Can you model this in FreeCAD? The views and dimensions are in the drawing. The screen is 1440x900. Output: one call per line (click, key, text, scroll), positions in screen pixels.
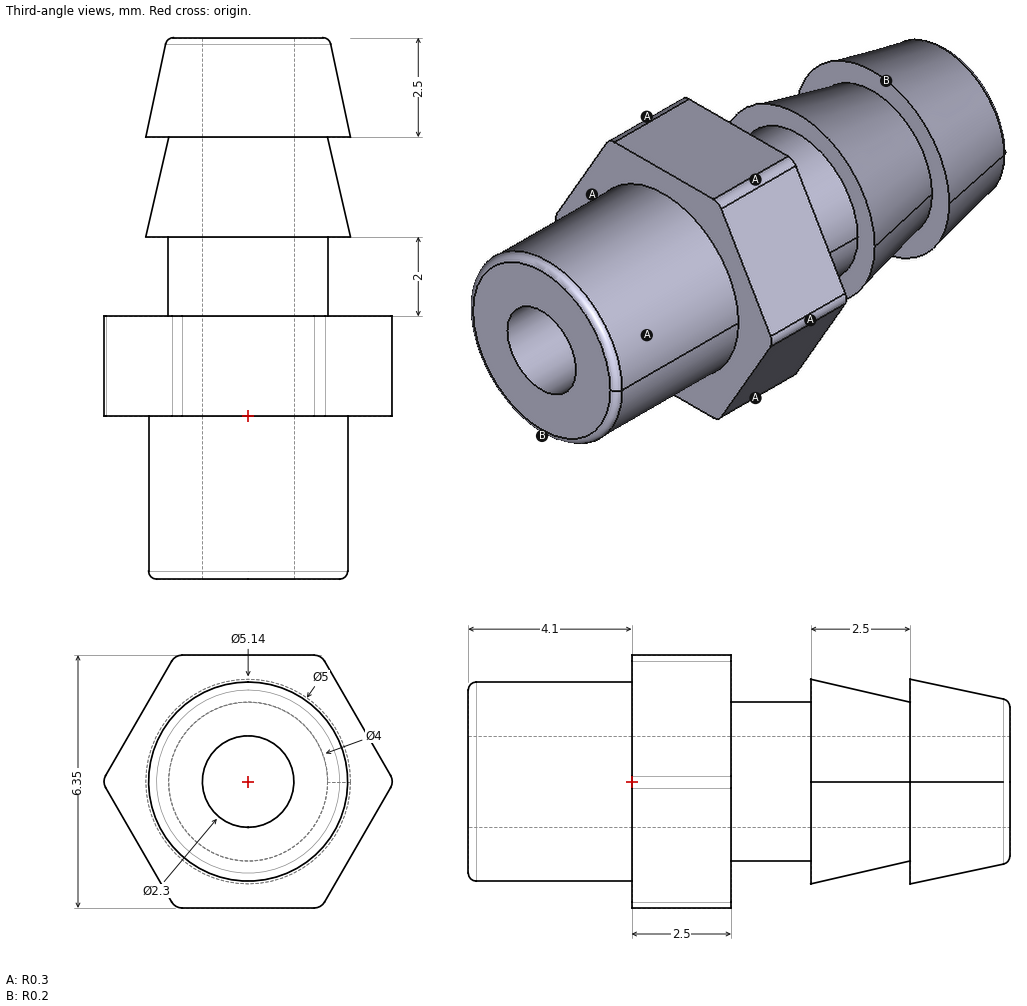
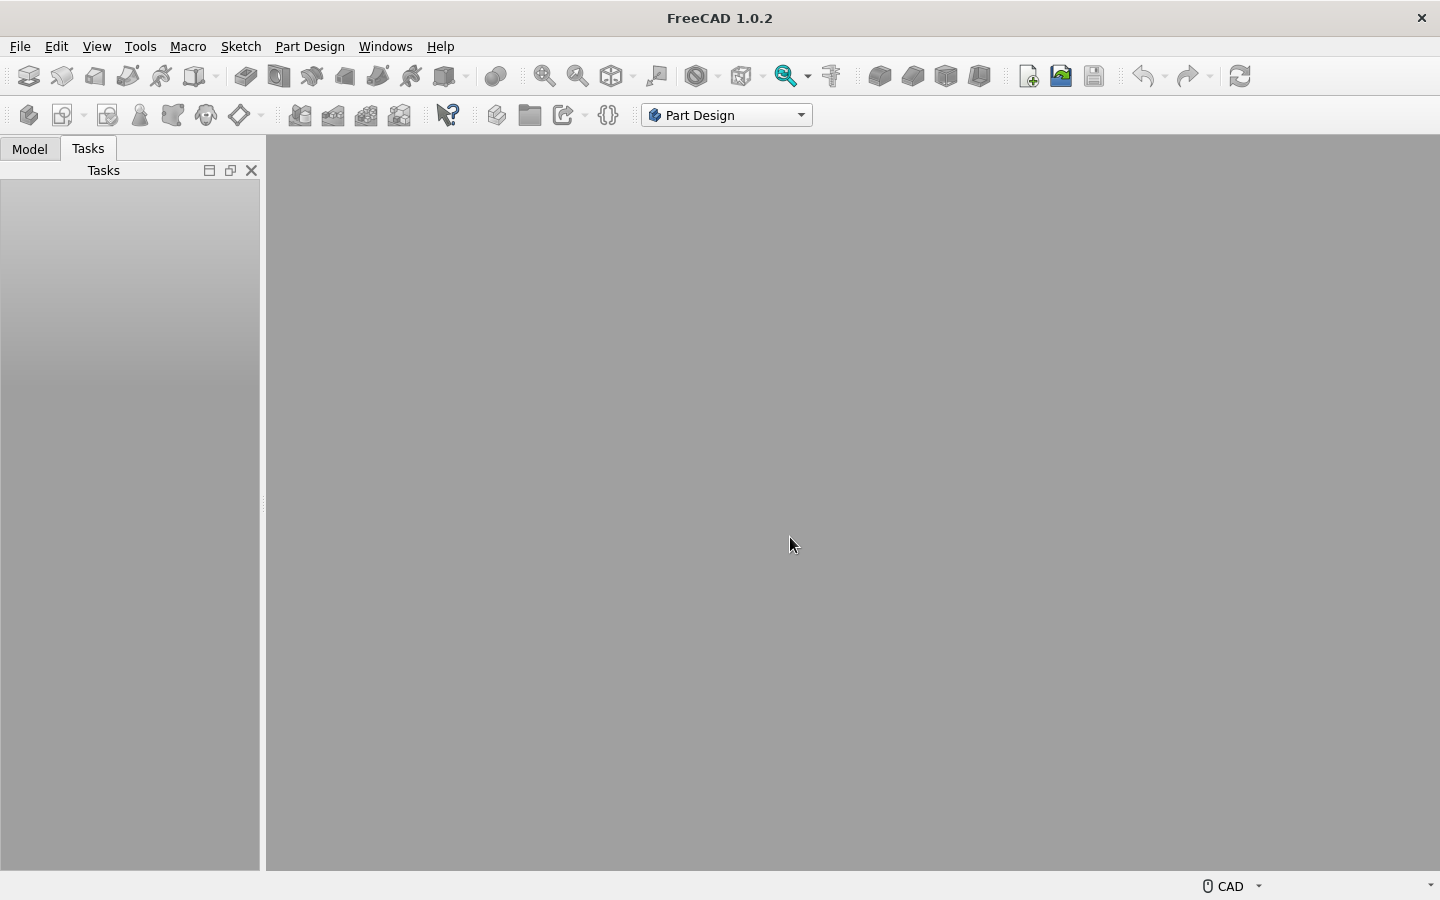
key(ctrl+n)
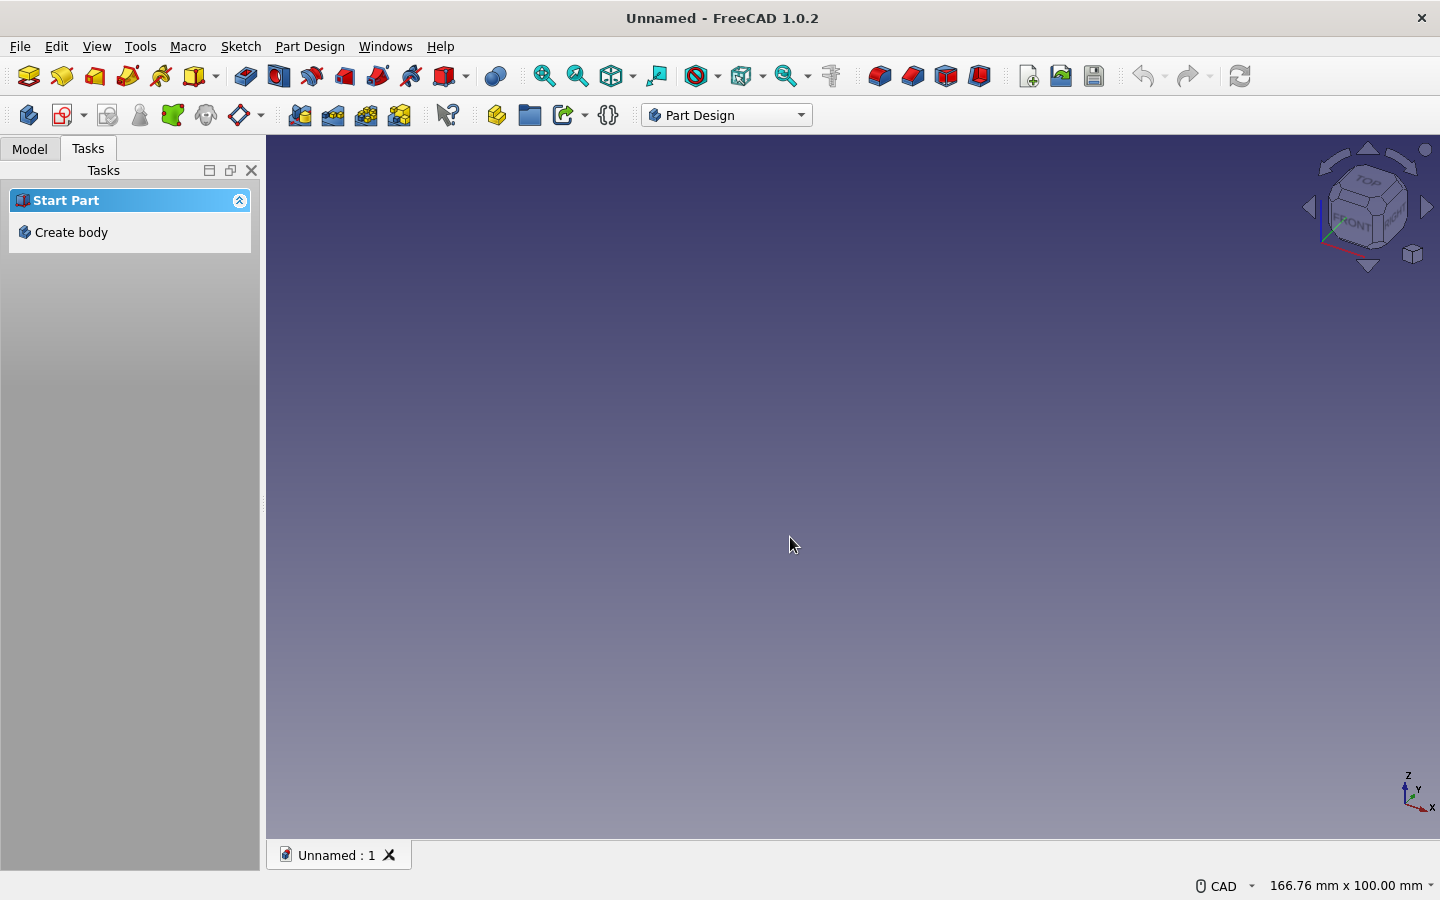
click(62, 116)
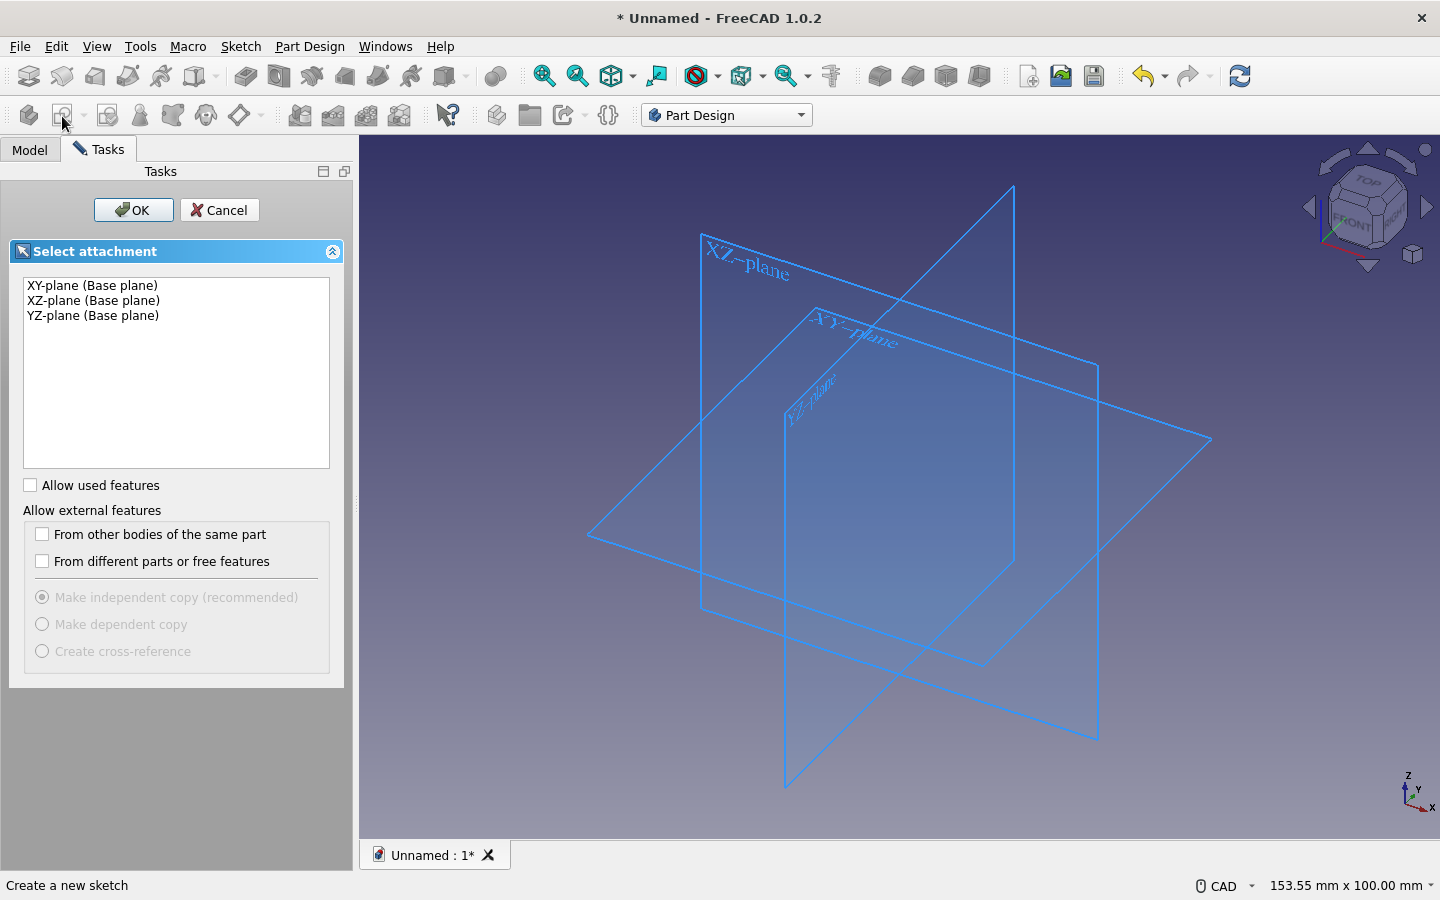
click(84, 300)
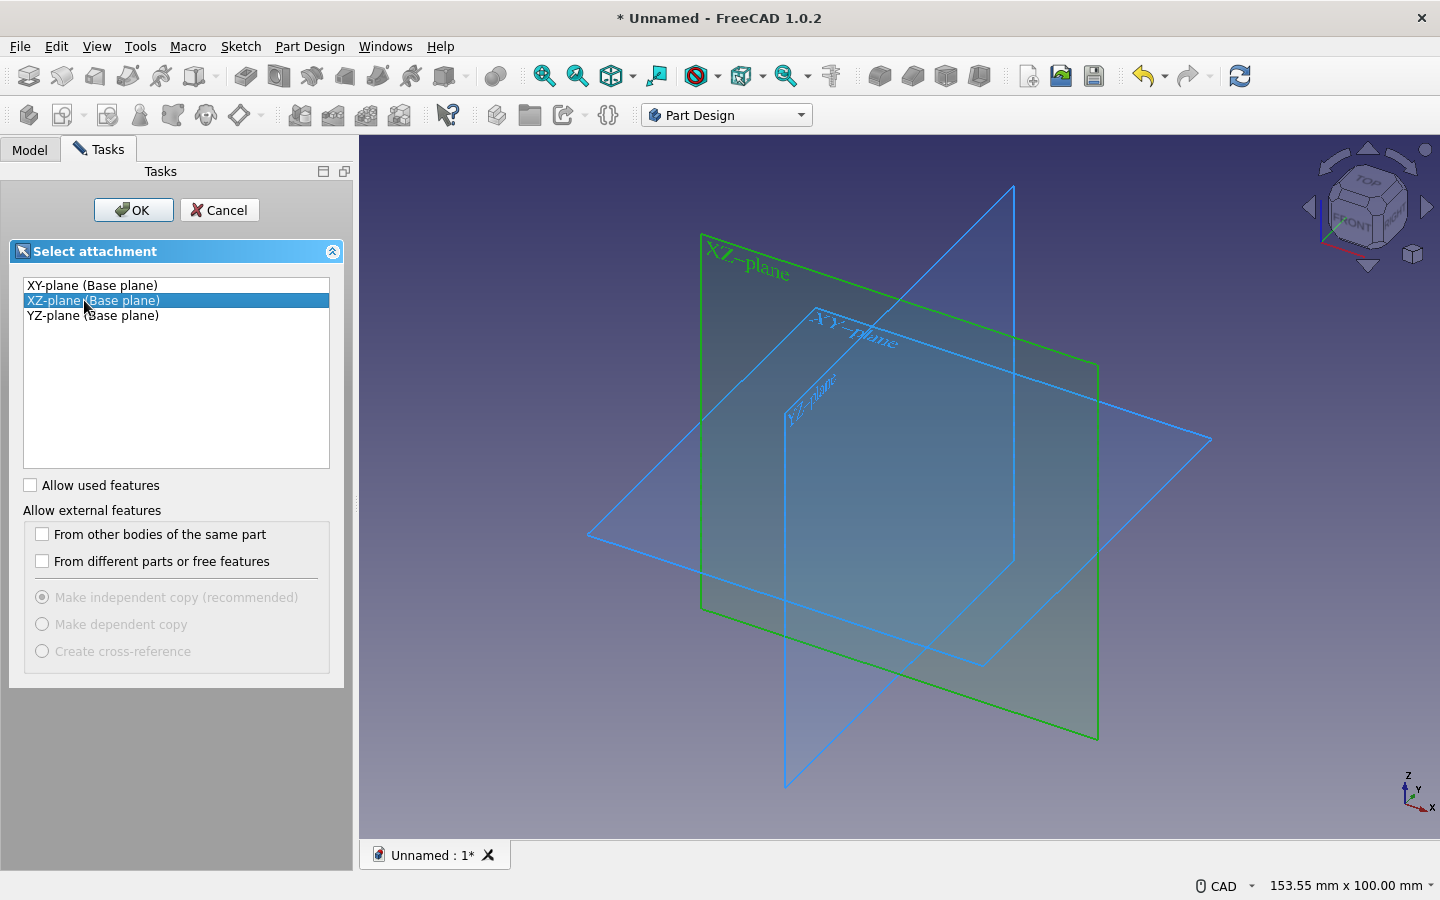
click(134, 210)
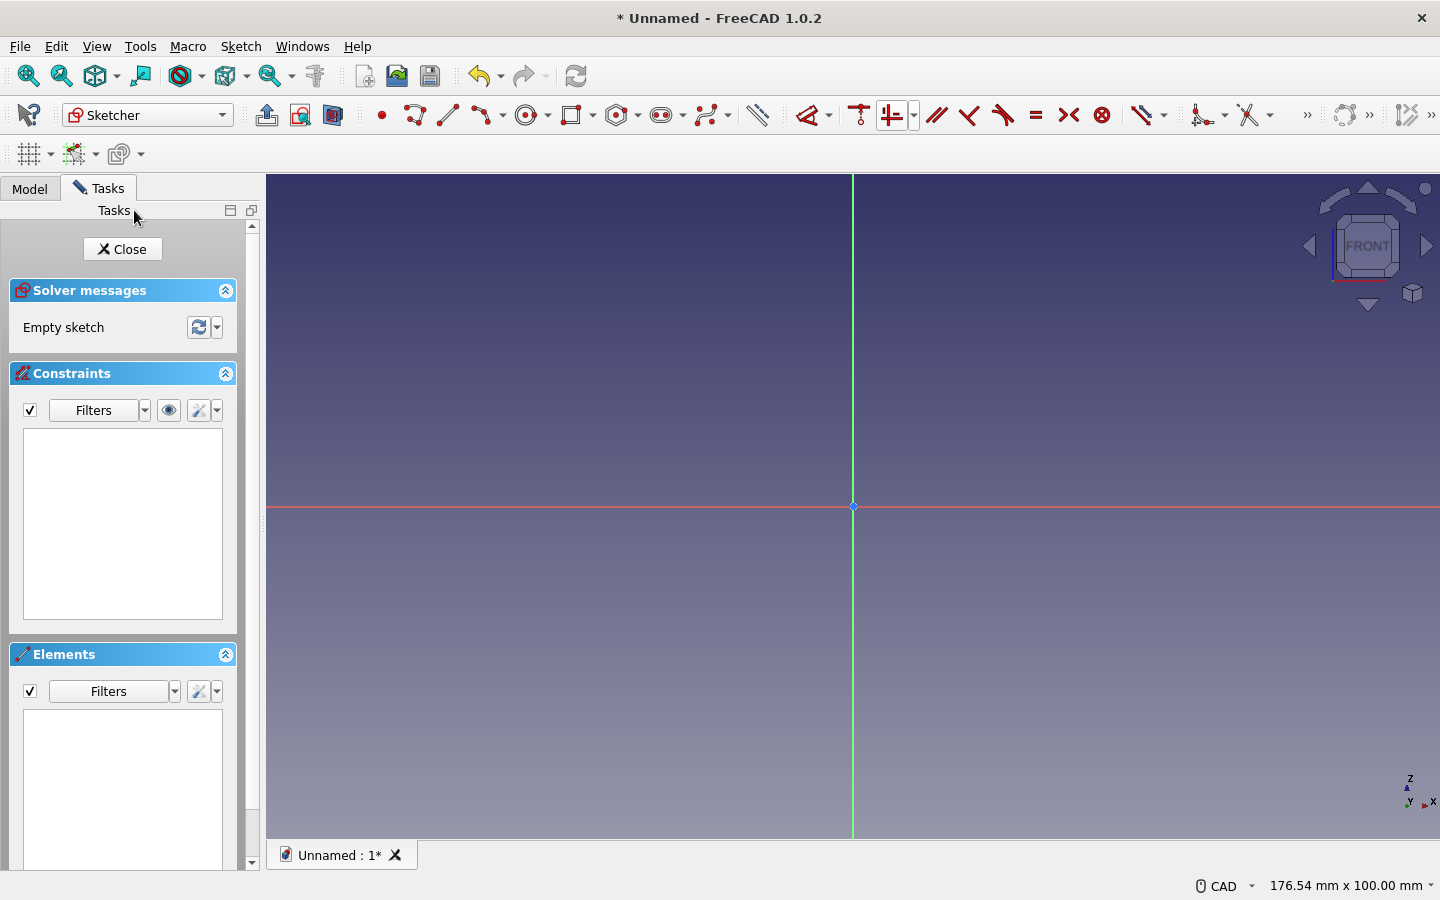
scroll(860, 506, up, 12)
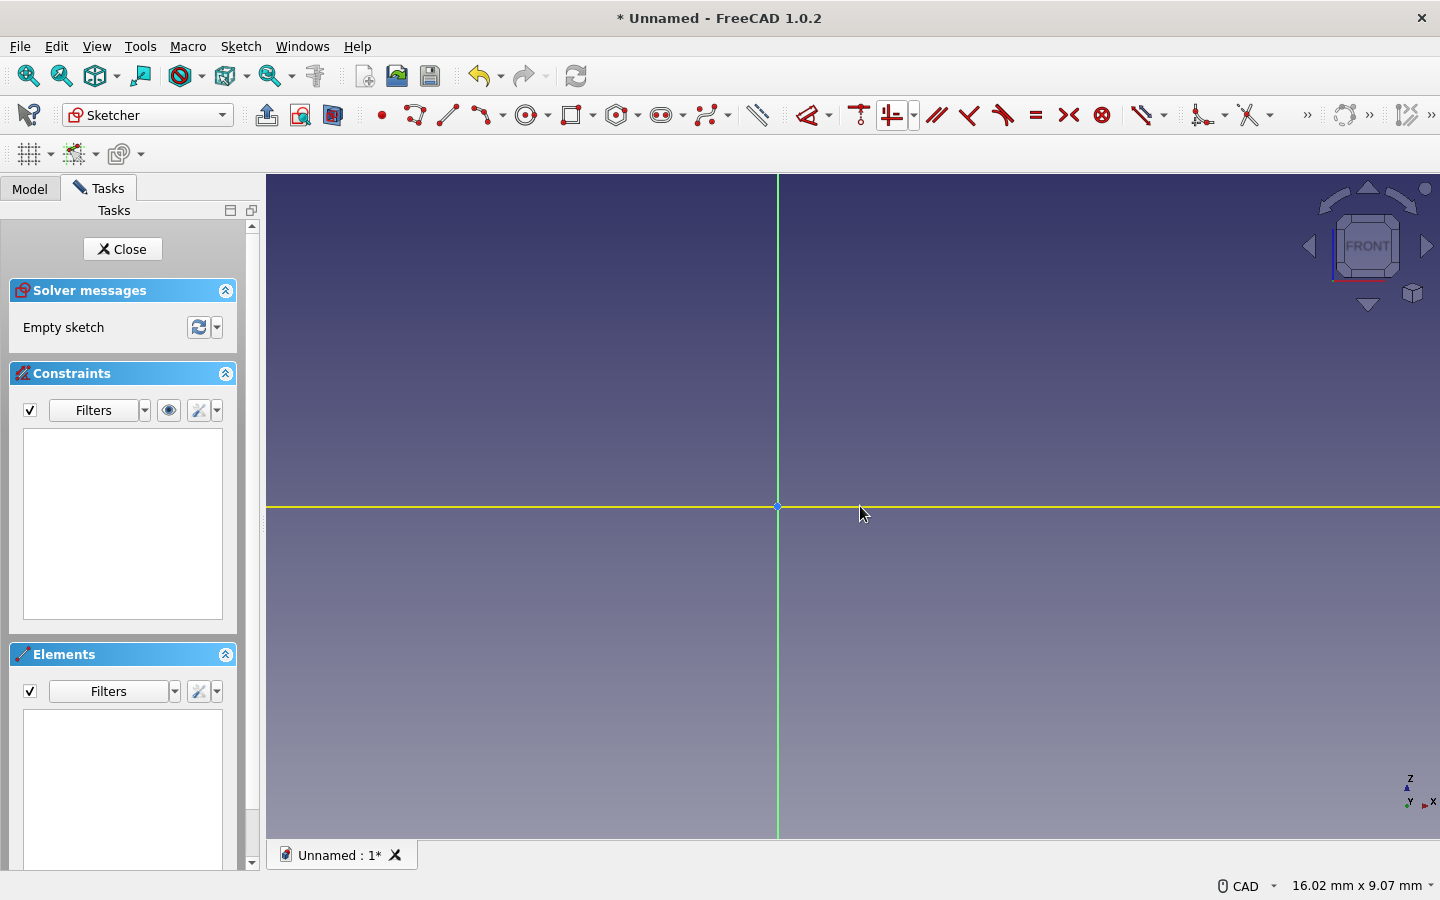
click(616, 116)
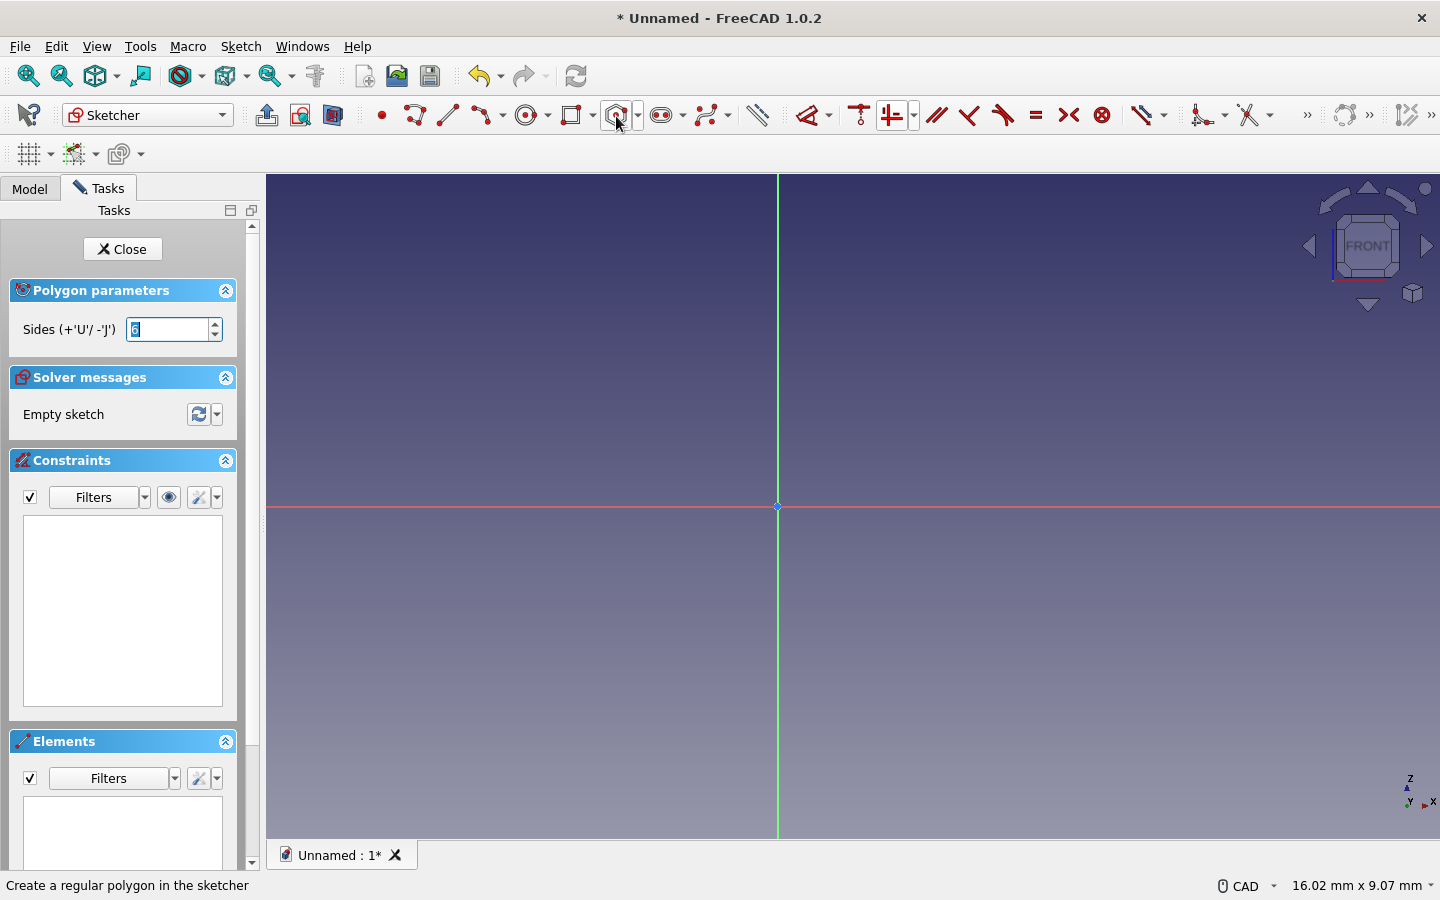
click(778, 506)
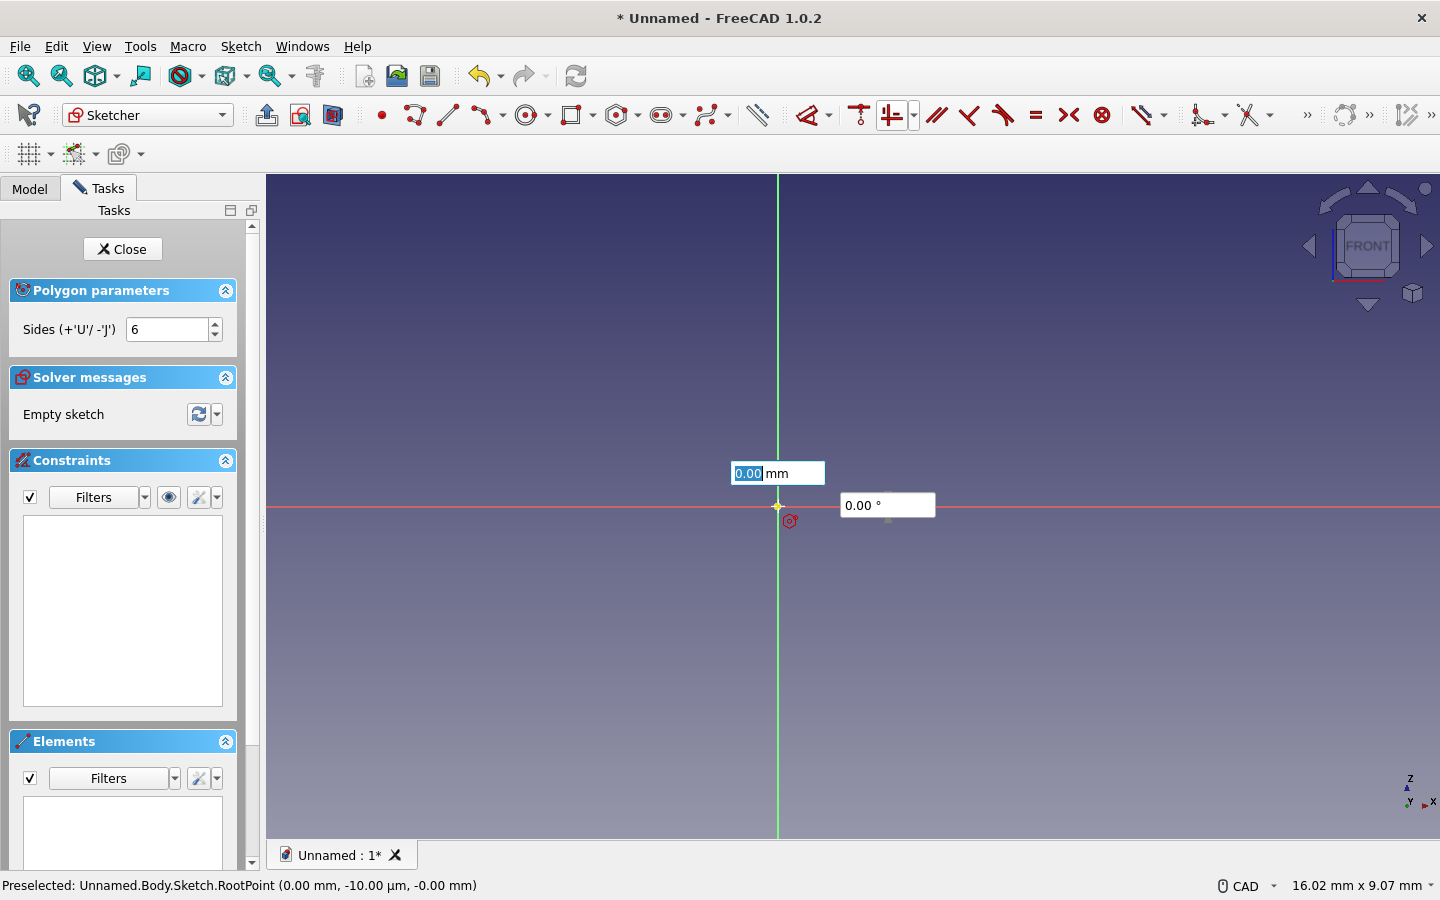
click(1047, 506)
key(Escape)